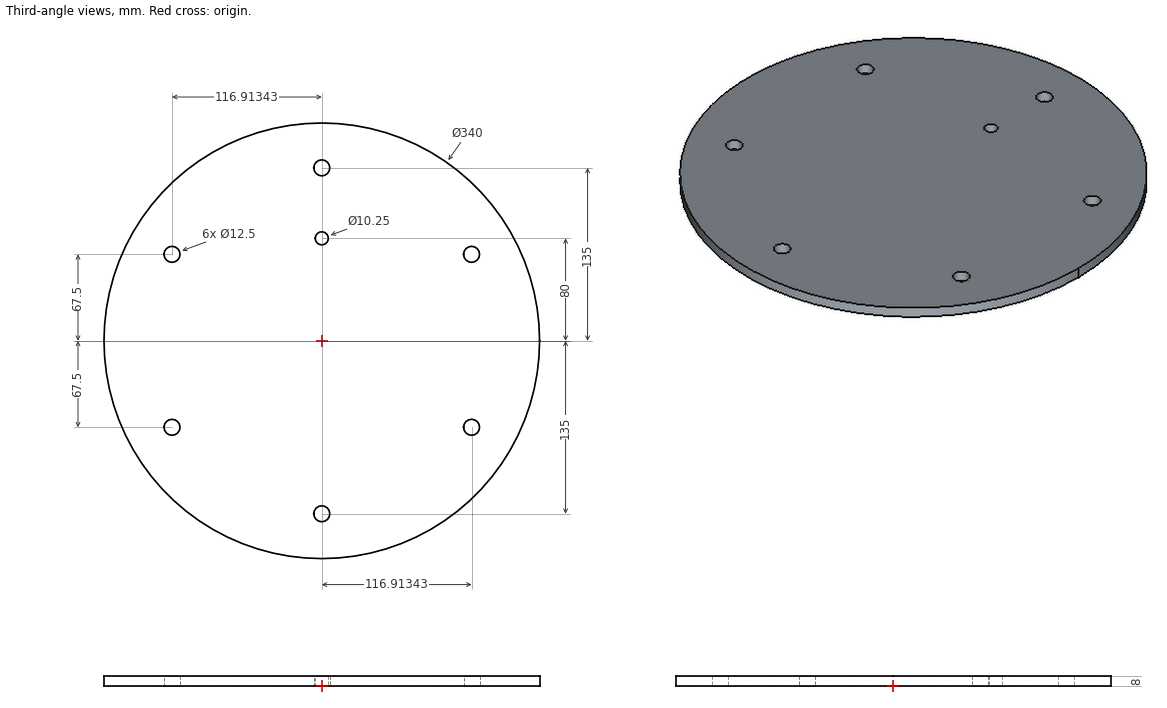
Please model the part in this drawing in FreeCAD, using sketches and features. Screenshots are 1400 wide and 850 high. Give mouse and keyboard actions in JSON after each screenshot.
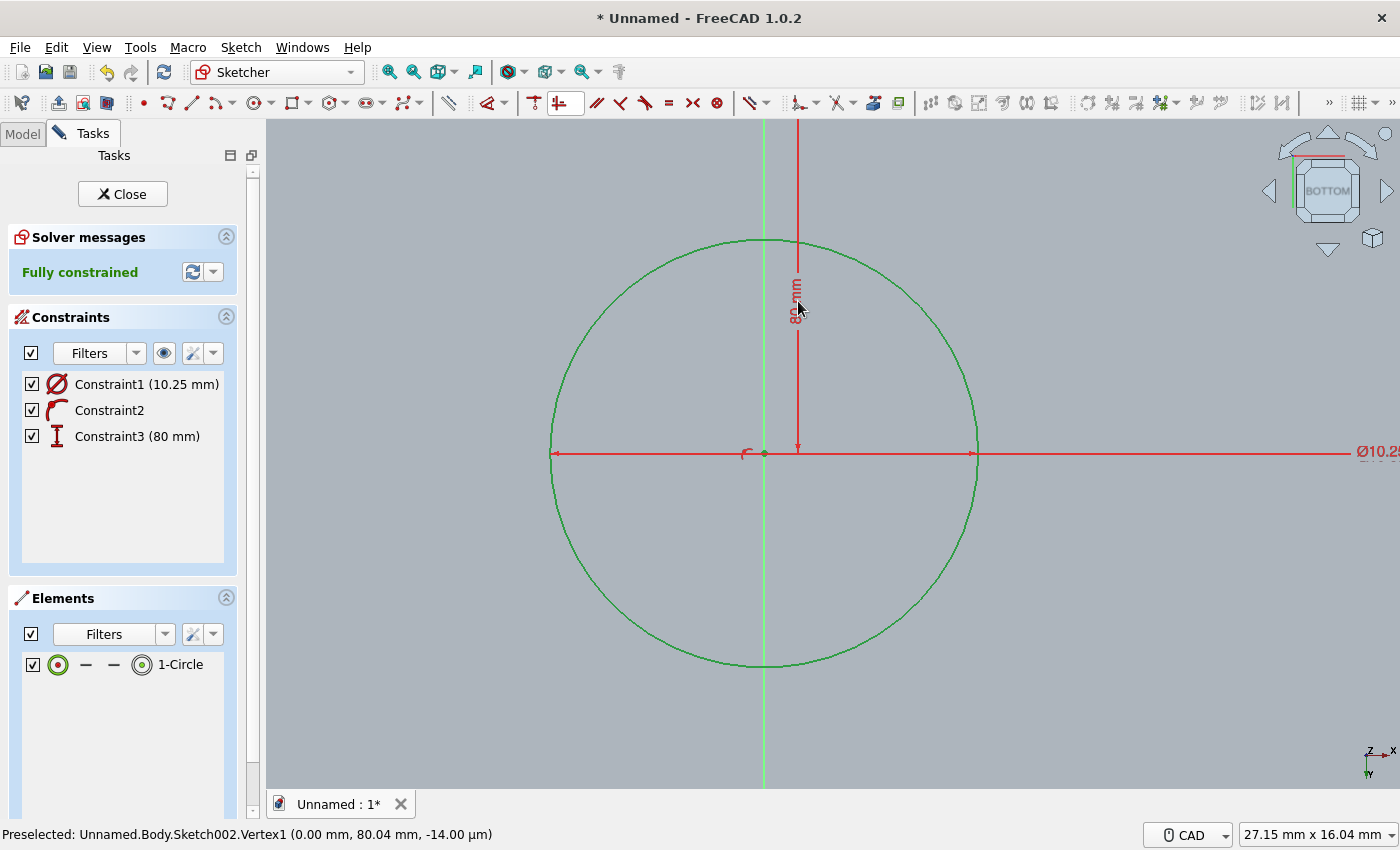
{"action": "left_click", "coordinate": [123, 194]}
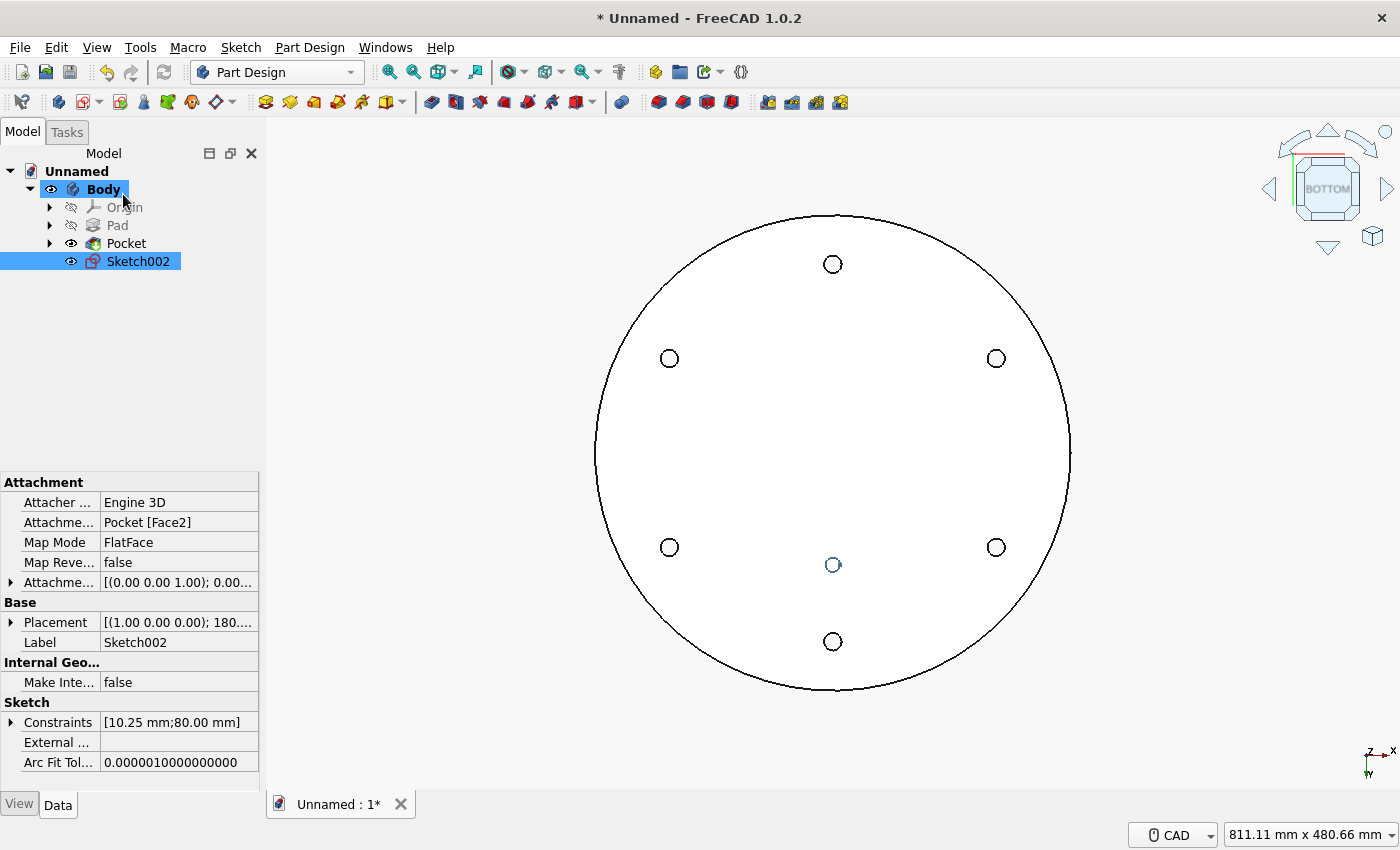
{"action": "left_click", "coordinate": [432, 102]}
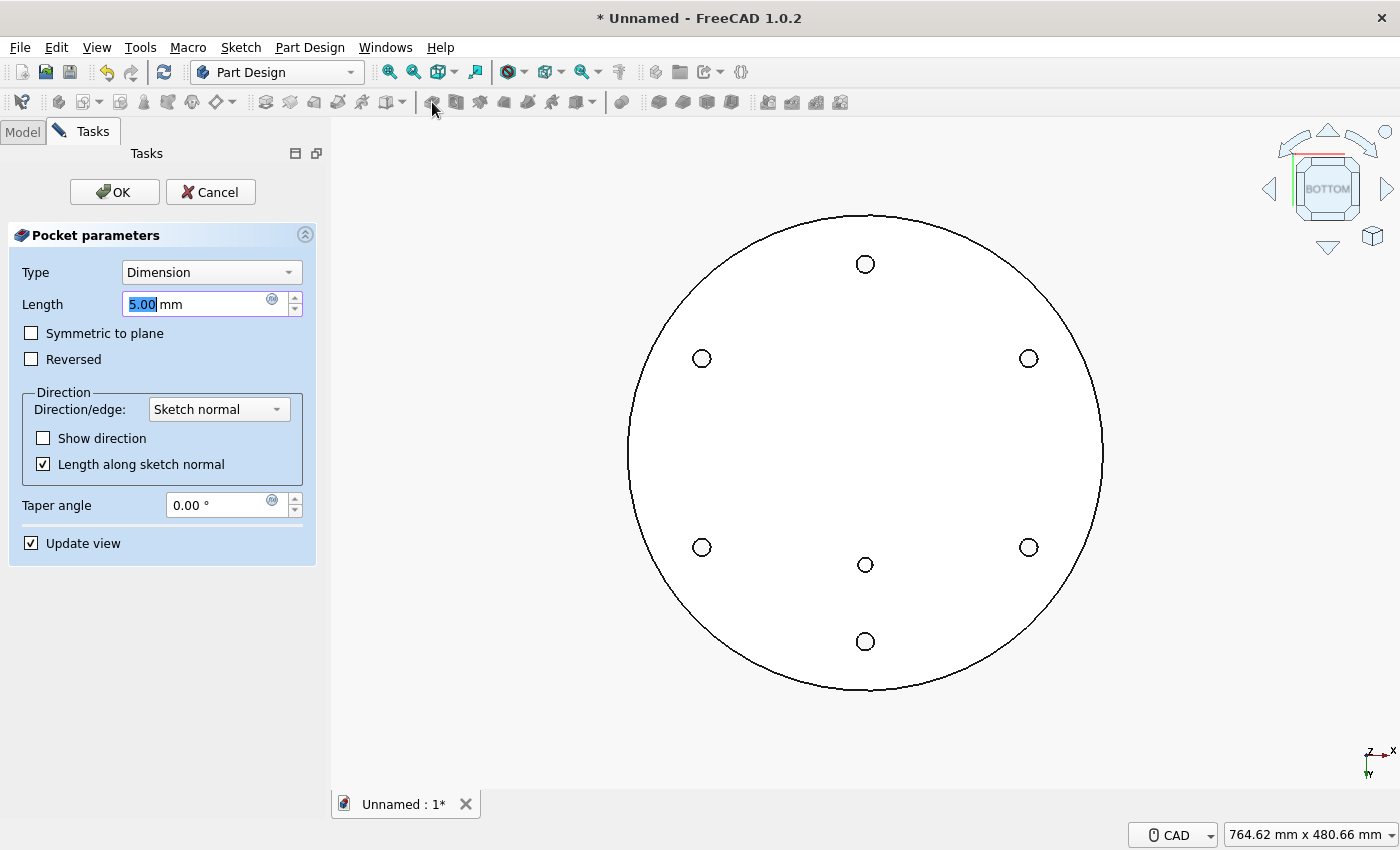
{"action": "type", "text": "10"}
{"action": "key", "text": "Tab"}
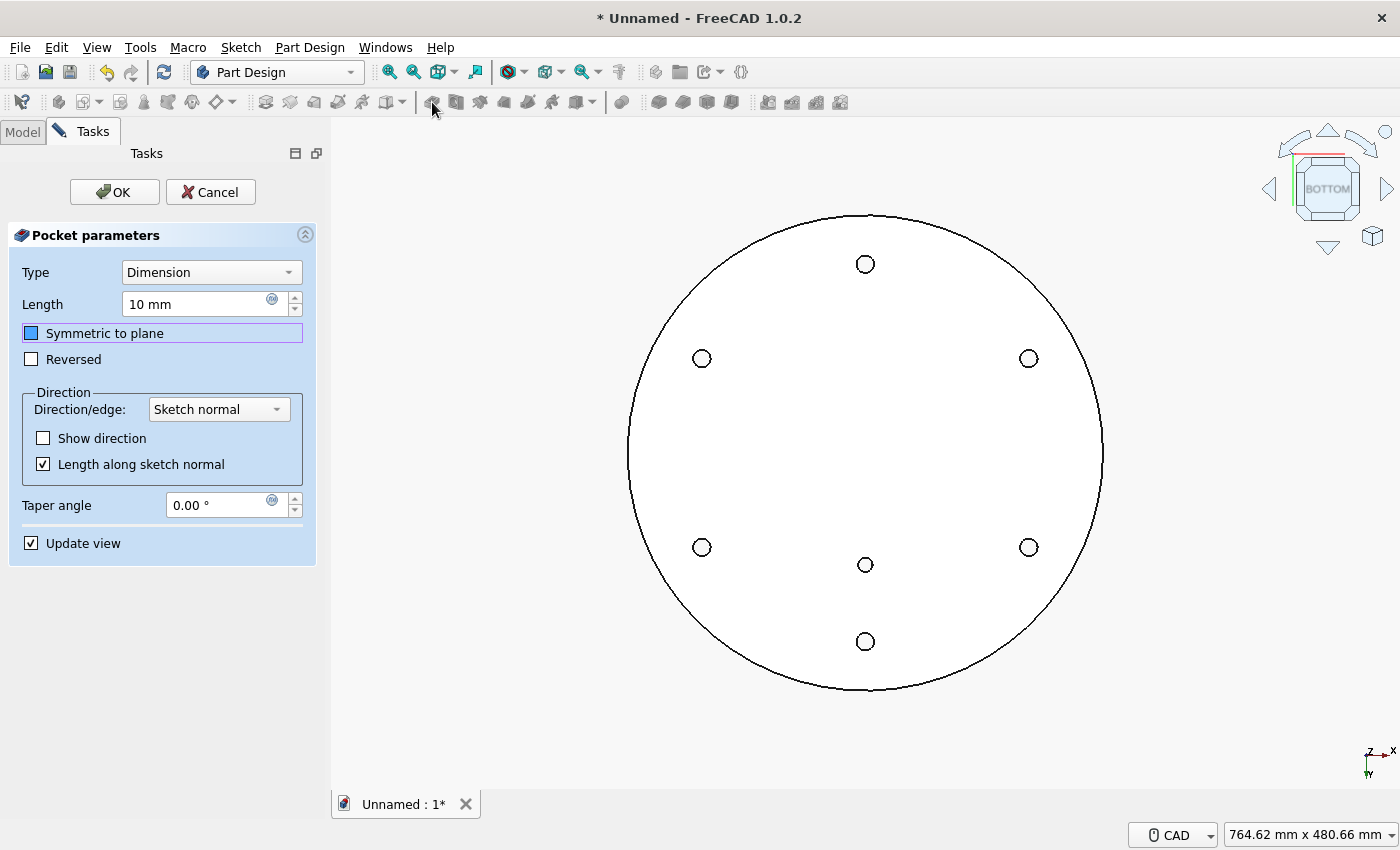
{"action": "left_click", "coordinate": [115, 192]}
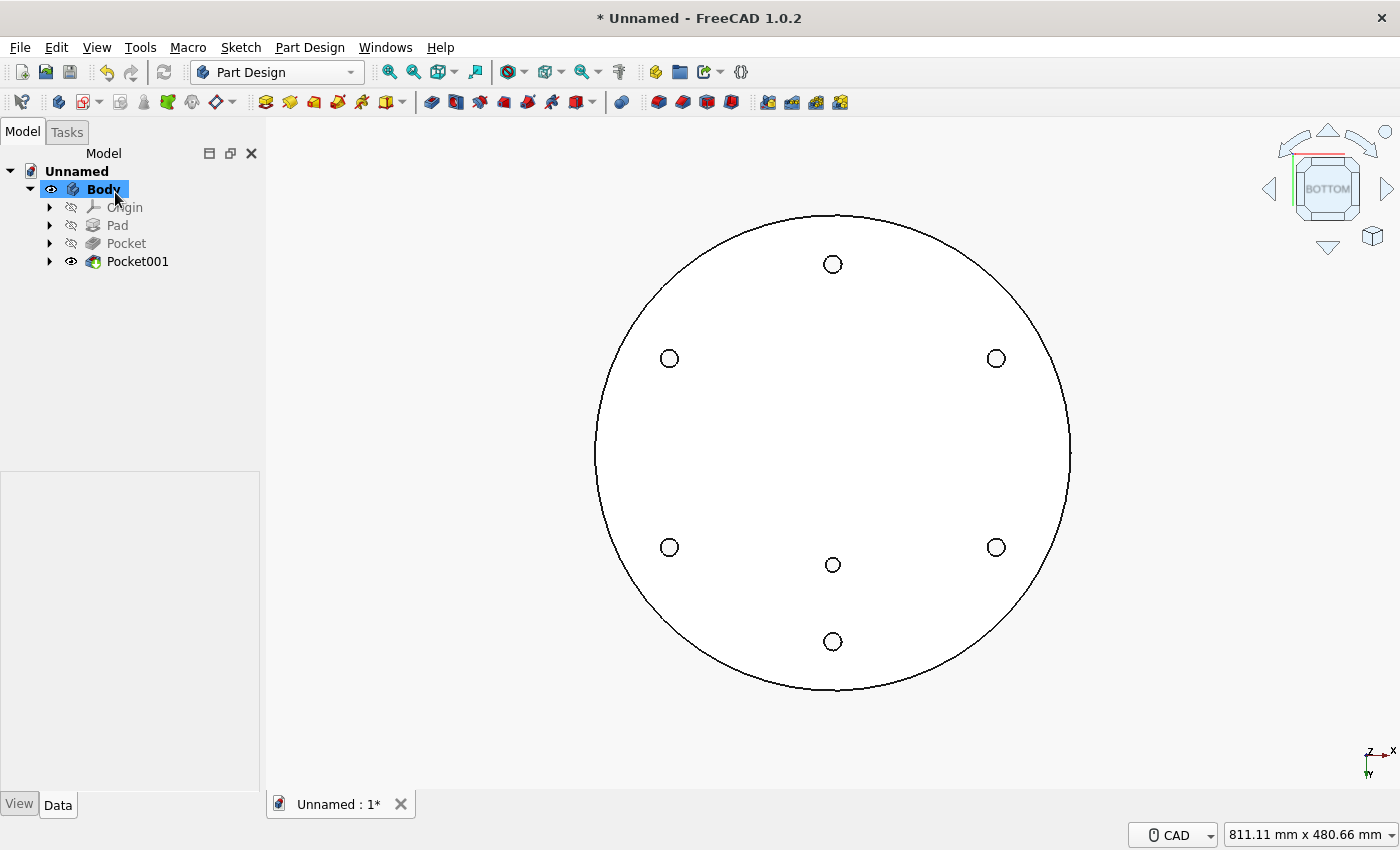
{"action": "key", "text": "0"}